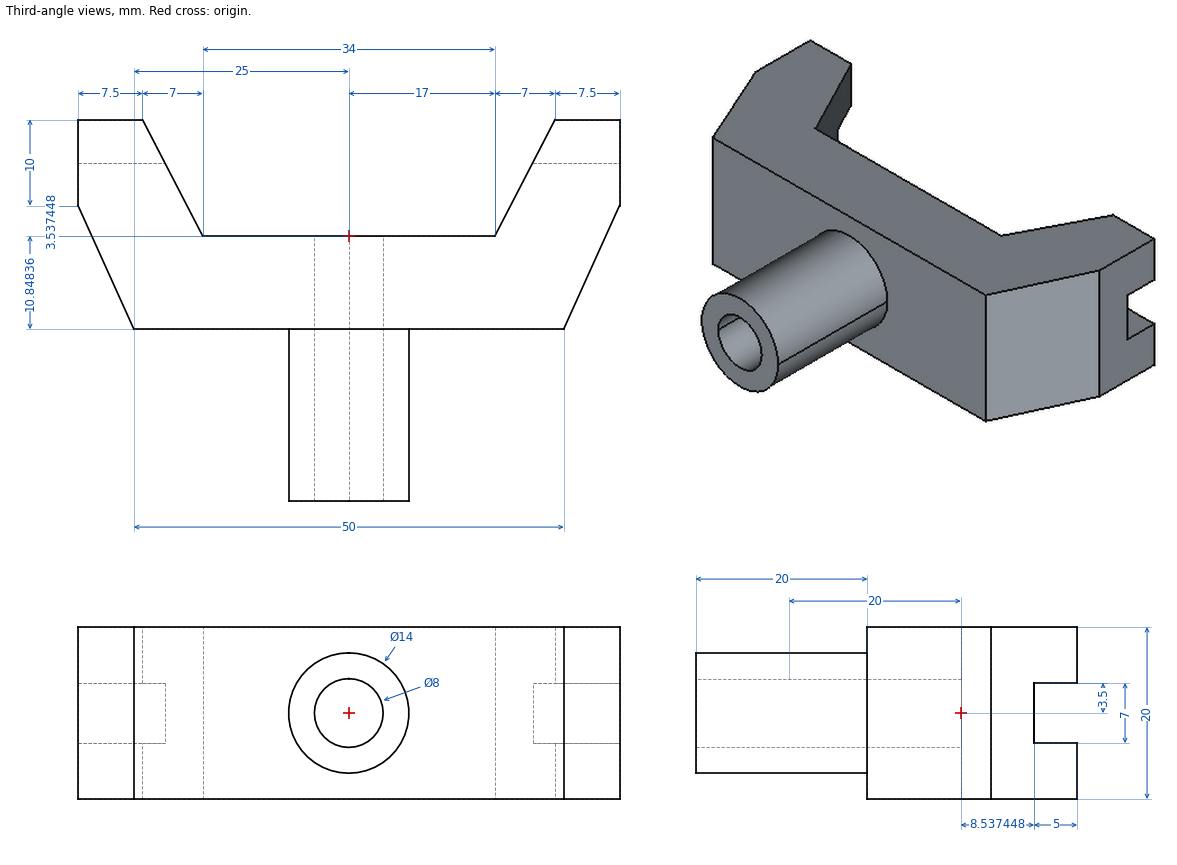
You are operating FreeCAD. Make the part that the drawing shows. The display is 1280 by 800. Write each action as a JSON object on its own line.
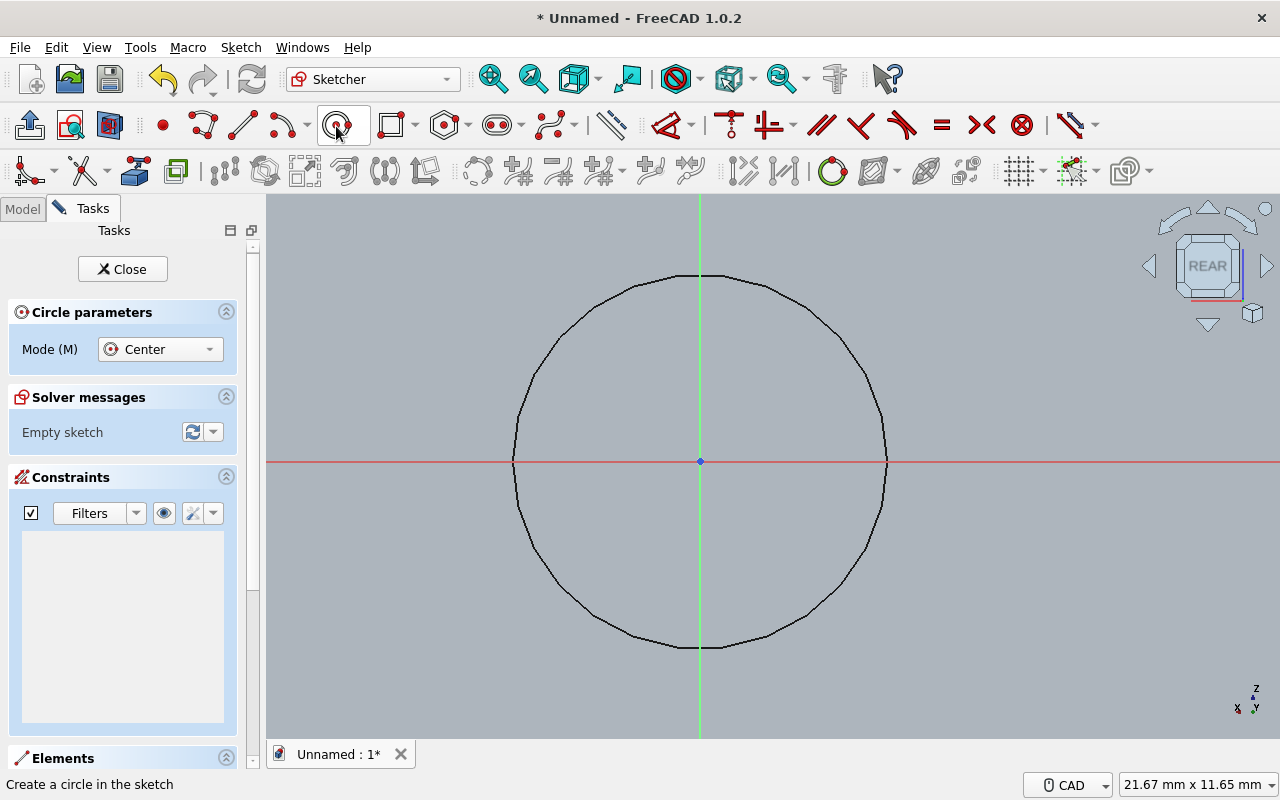
{"action": "left_click", "coordinate": [700, 462]}
{"action": "mouse_move", "coordinate": [832, 329]}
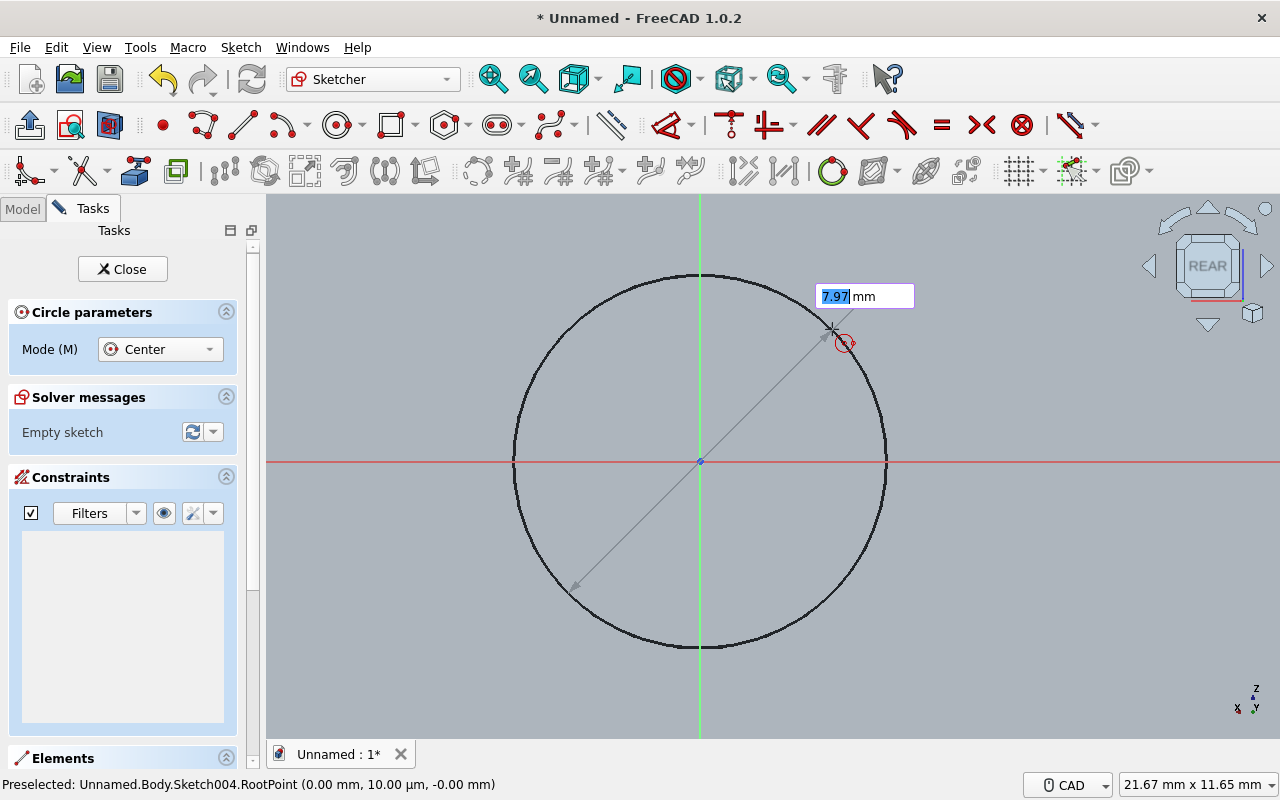
{"action": "type", "text": "8"}
{"action": "key", "text": "Return"}
{"action": "key", "text": "Escape"}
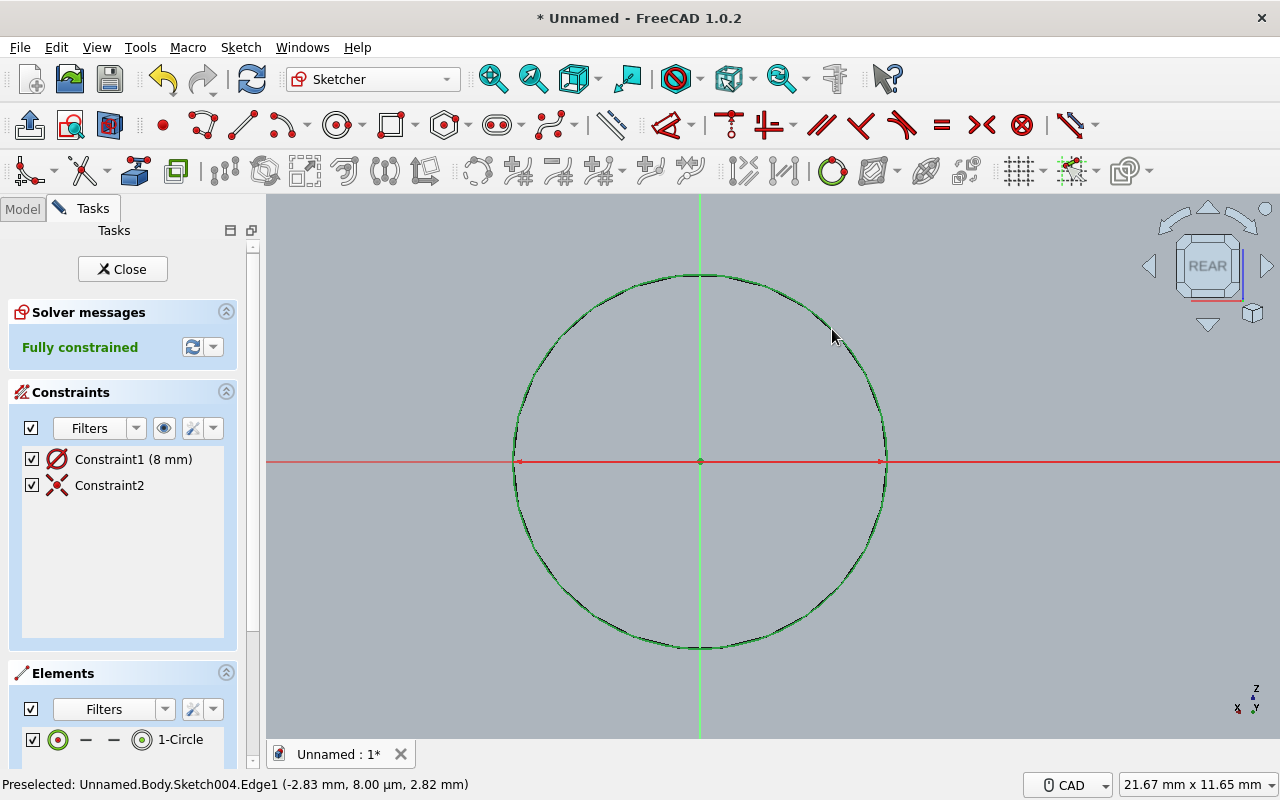
{"action": "left_click", "coordinate": [123, 269]}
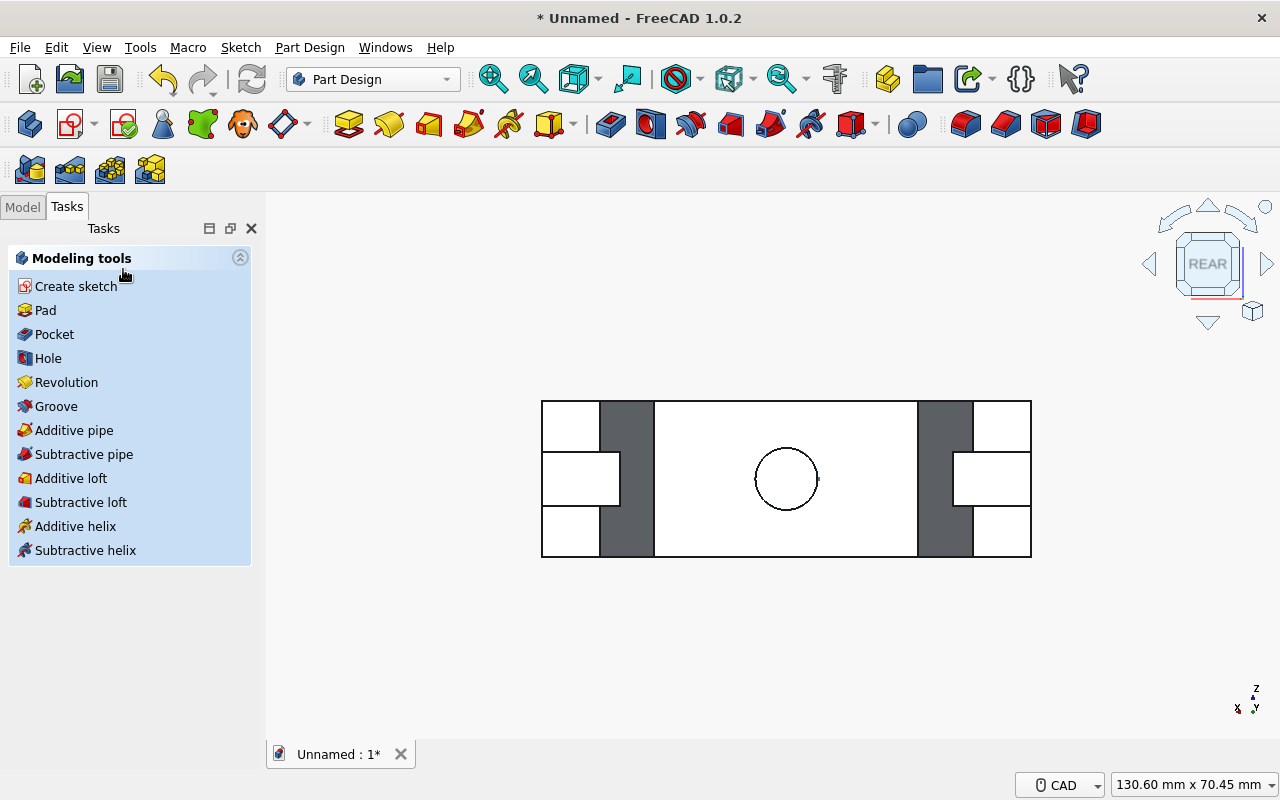
{"action": "left_click", "coordinate": [612, 124]}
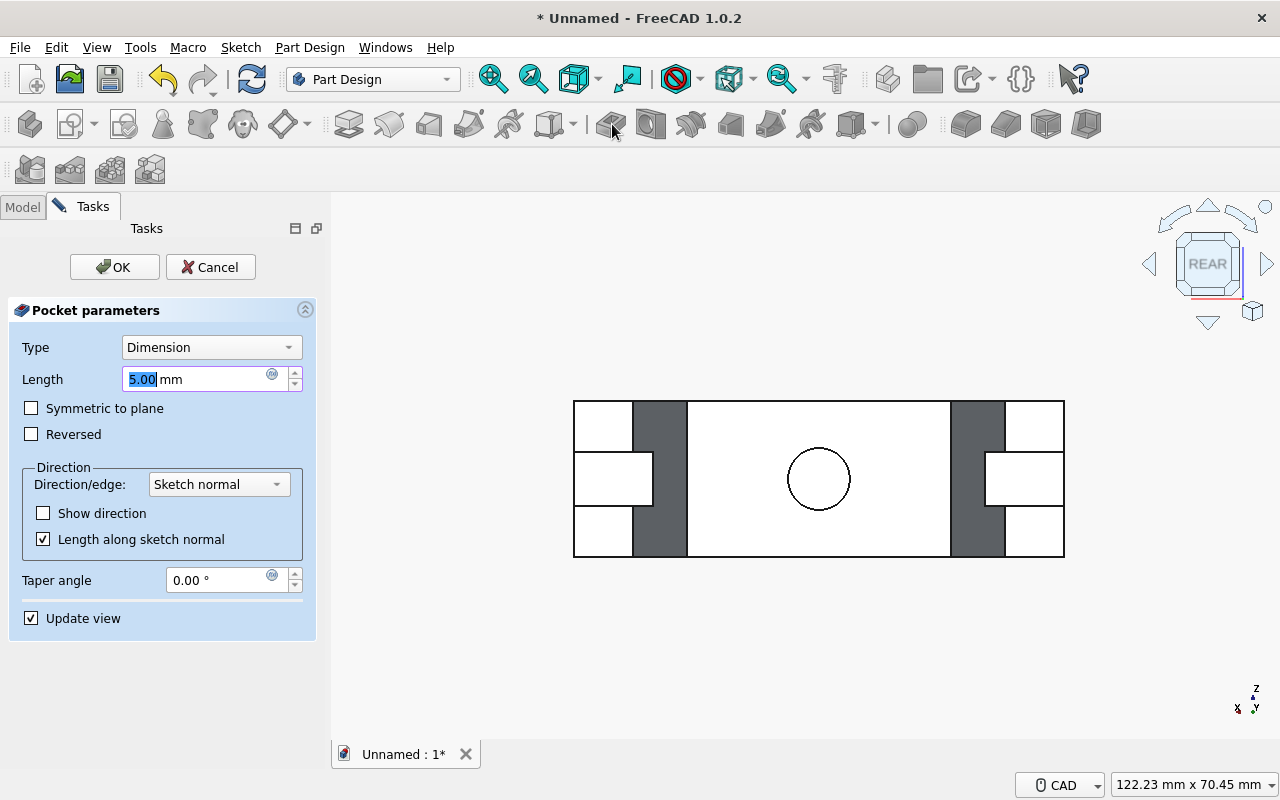
{"action": "left_click", "coordinate": [212, 348]}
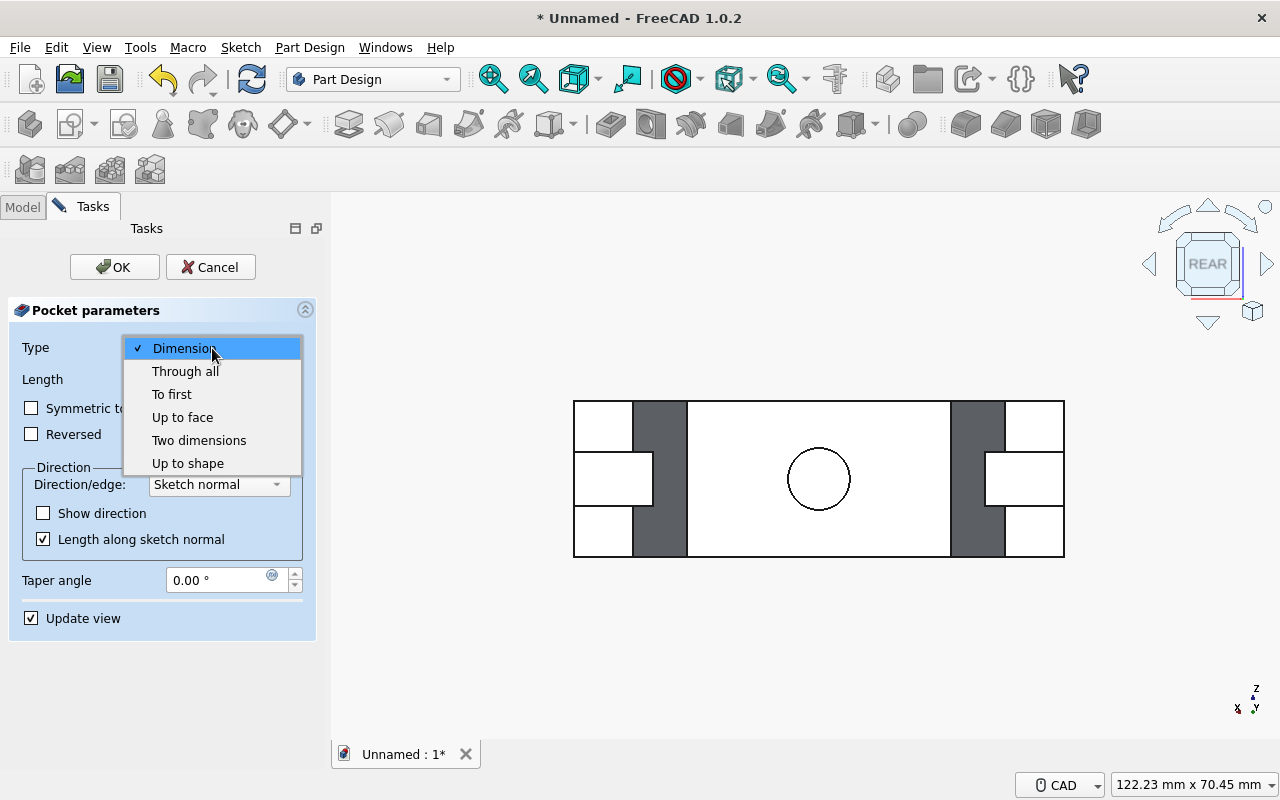
{"action": "left_click", "coordinate": [212, 372]}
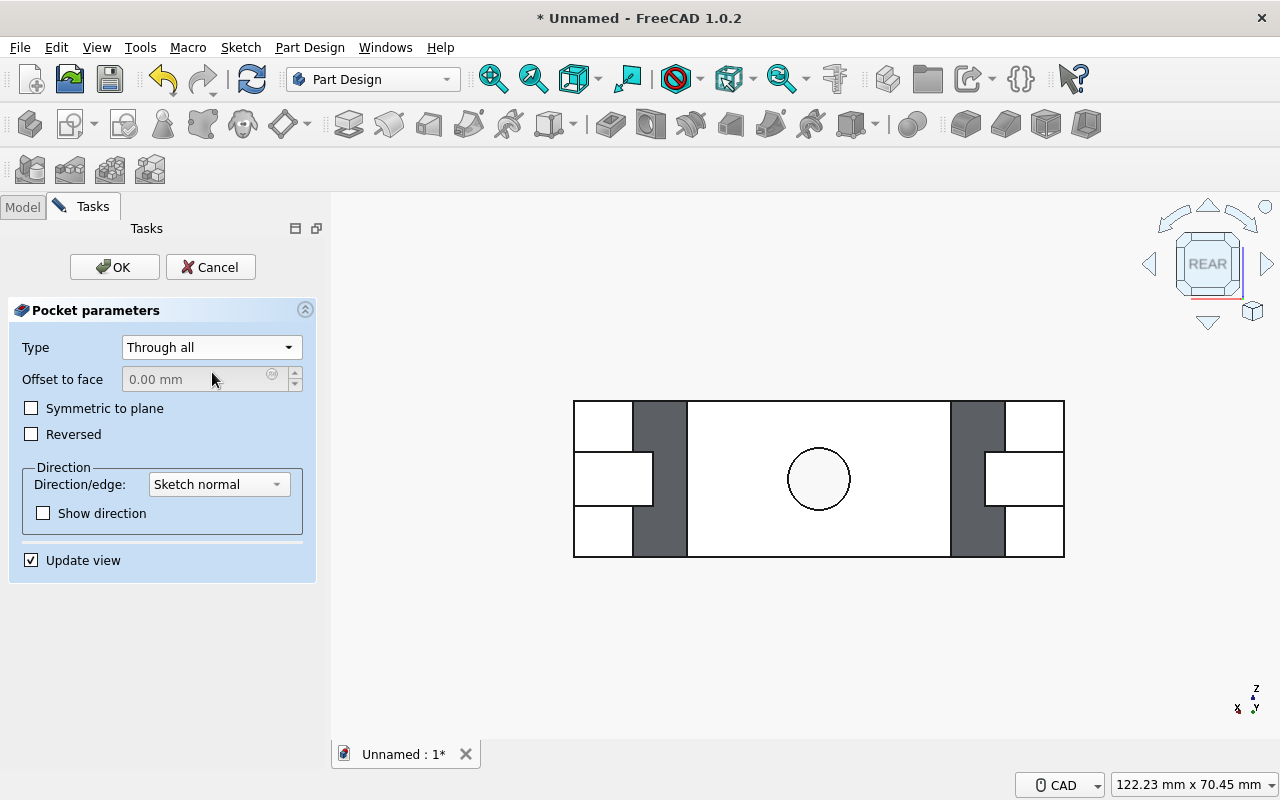
{"action": "left_click", "coordinate": [115, 267]}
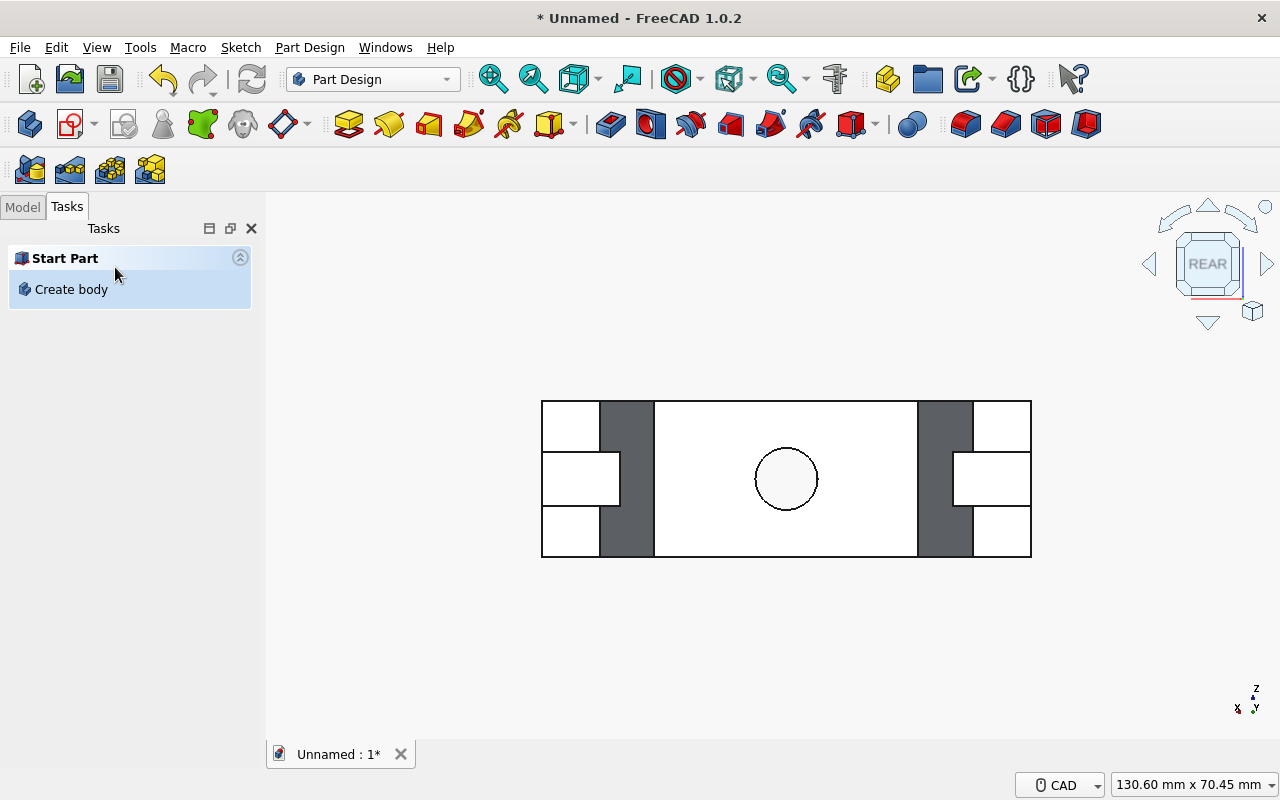
{"action": "key", "text": "0"}